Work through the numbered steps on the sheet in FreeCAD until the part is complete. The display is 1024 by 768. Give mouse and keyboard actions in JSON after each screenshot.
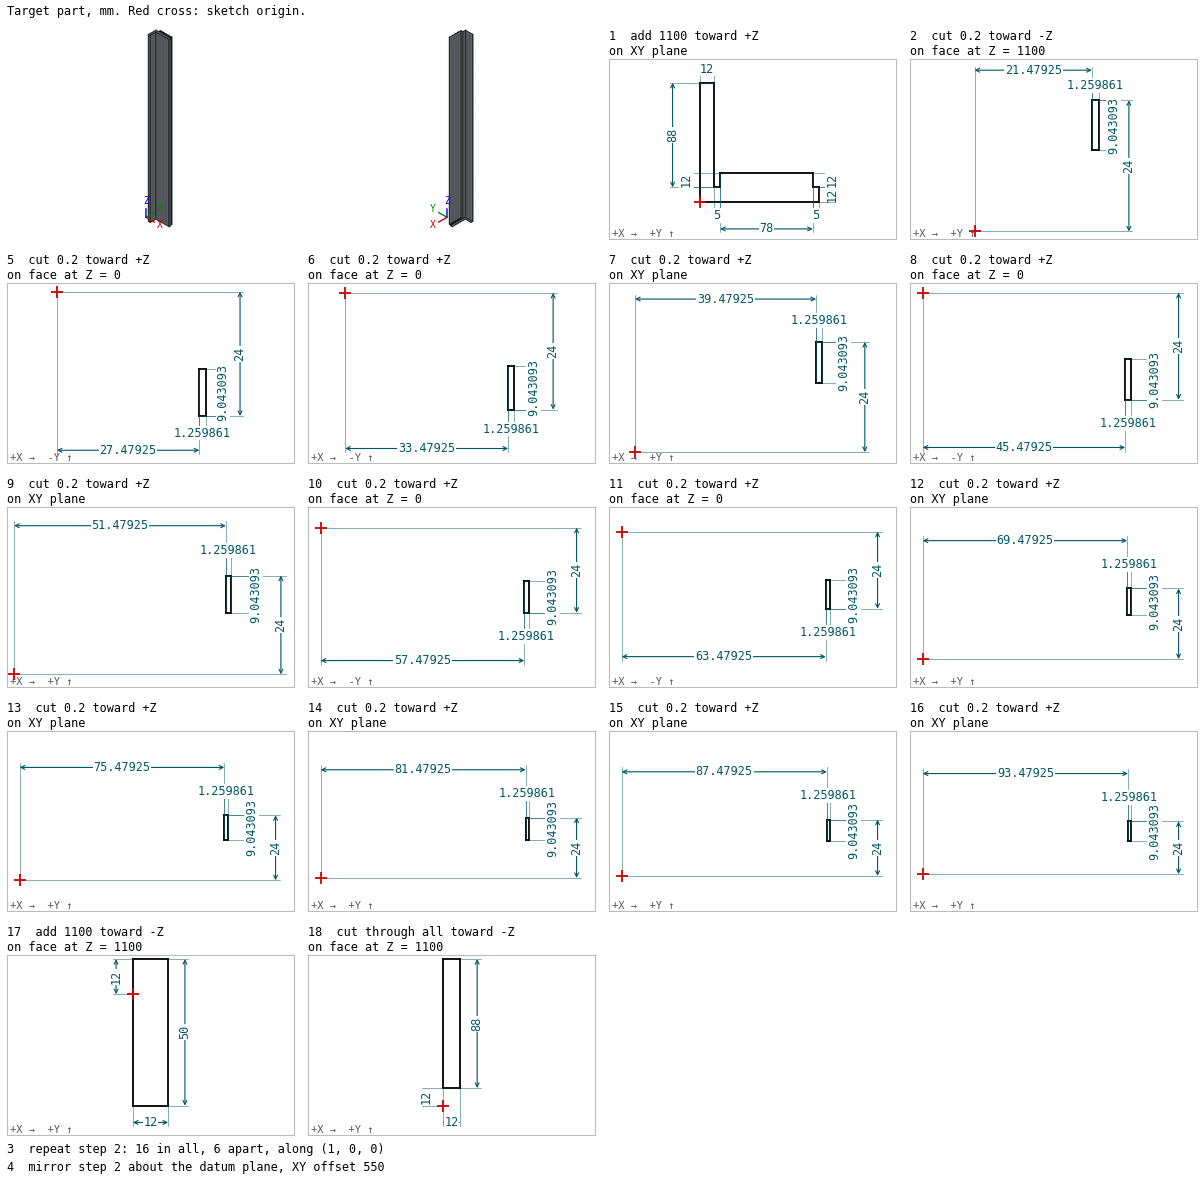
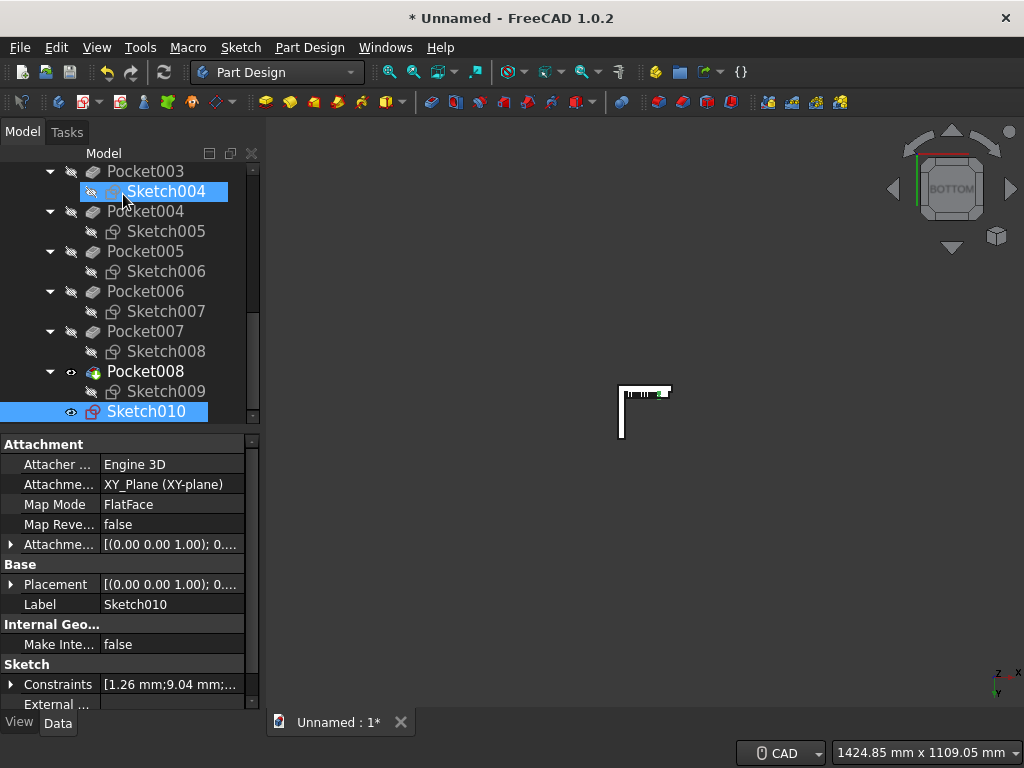
{"action": "left_click", "coordinate": [432, 102]}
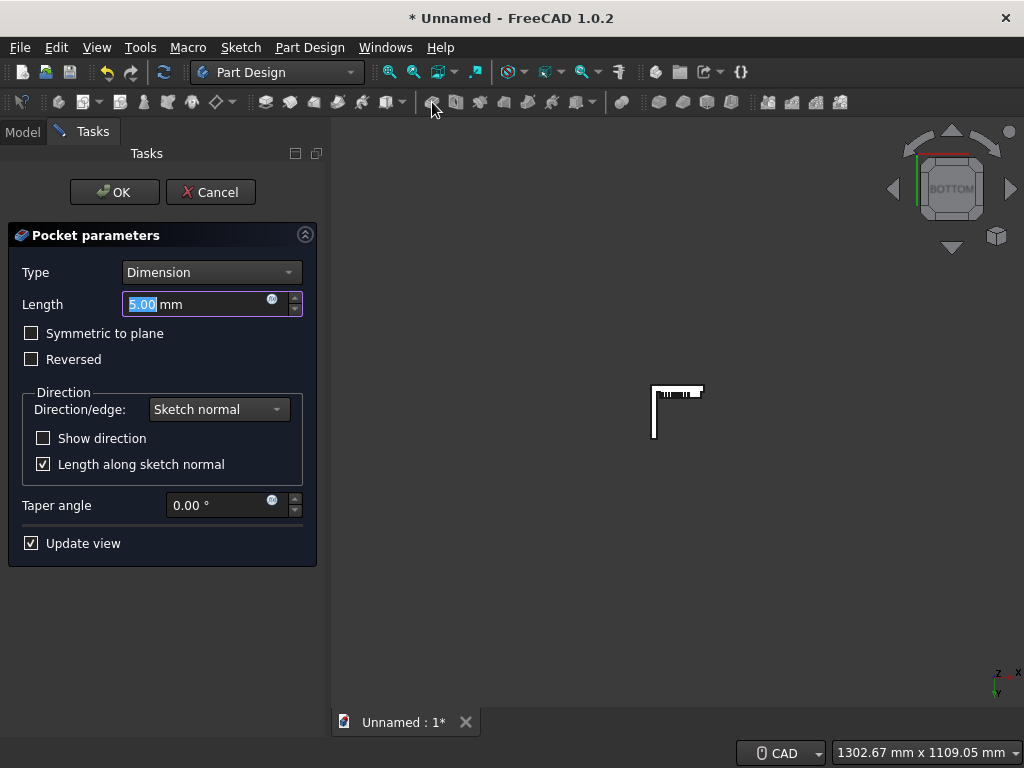
{"action": "type", "text": "0.2"}
{"action": "key", "text": "Tab"}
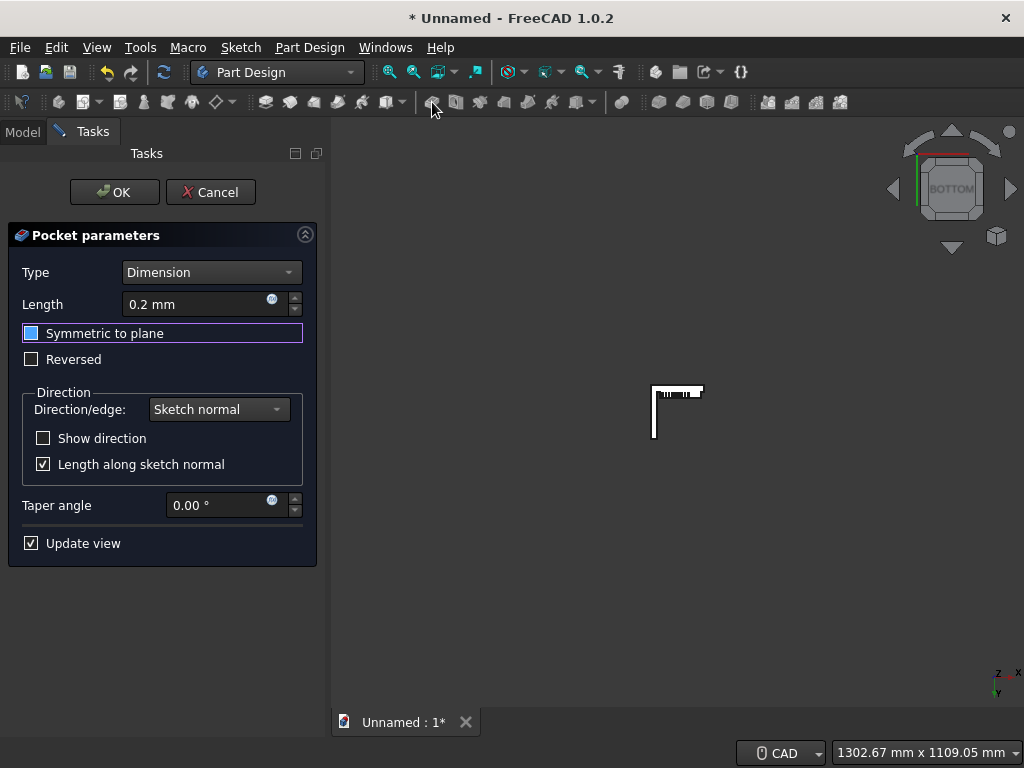
{"action": "left_click", "coordinate": [30, 359]}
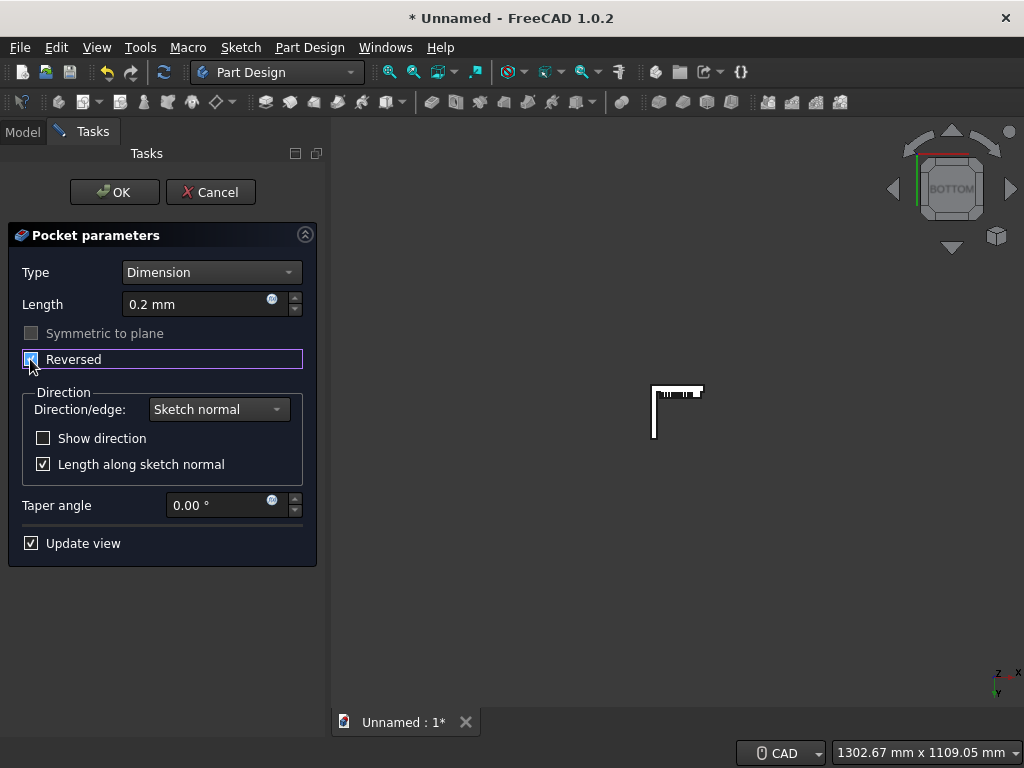
{"action": "left_click", "coordinate": [115, 192]}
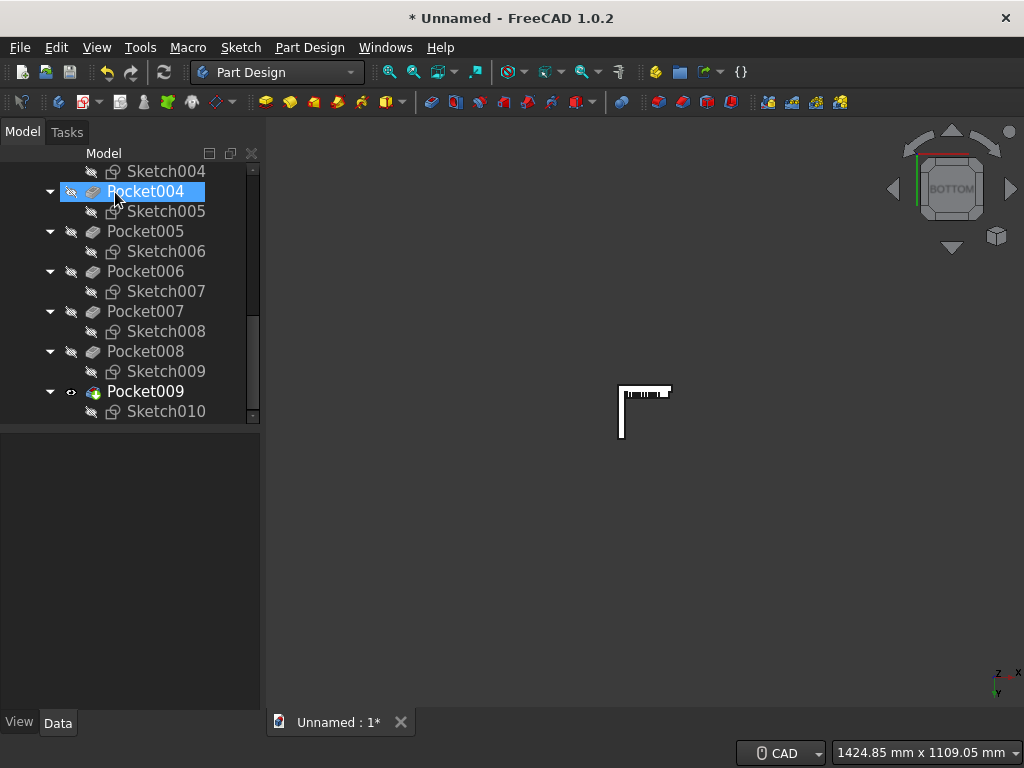
{"action": "left_click", "coordinate": [390, 72]}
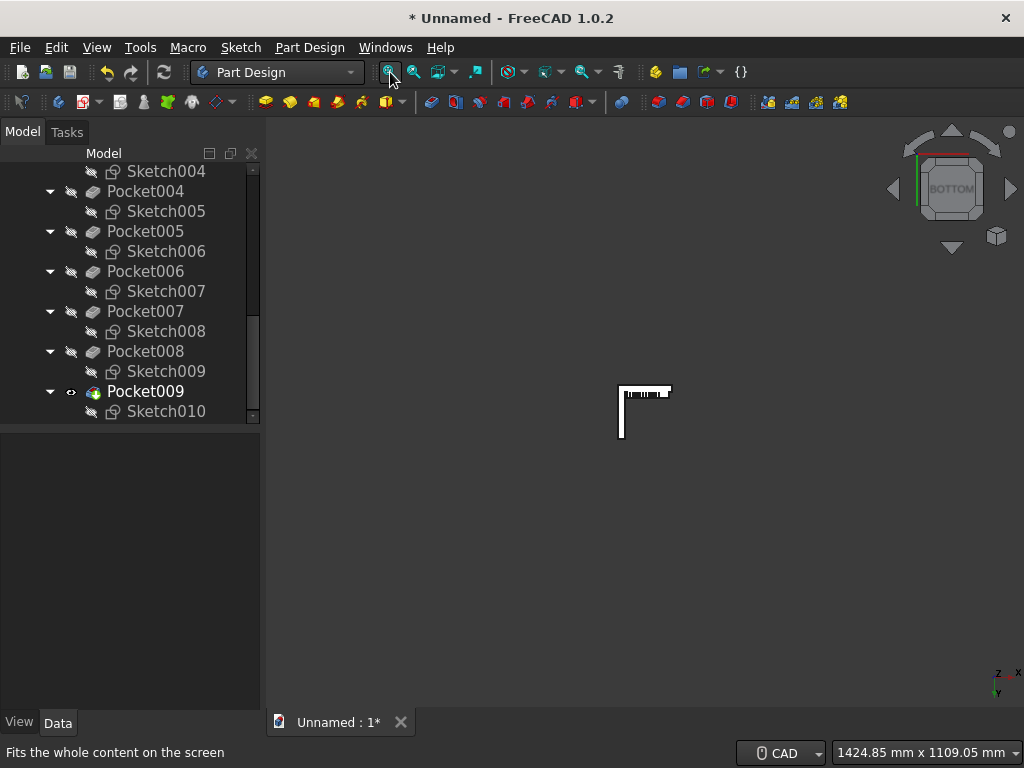
{"action": "left_click", "coordinate": [84, 102]}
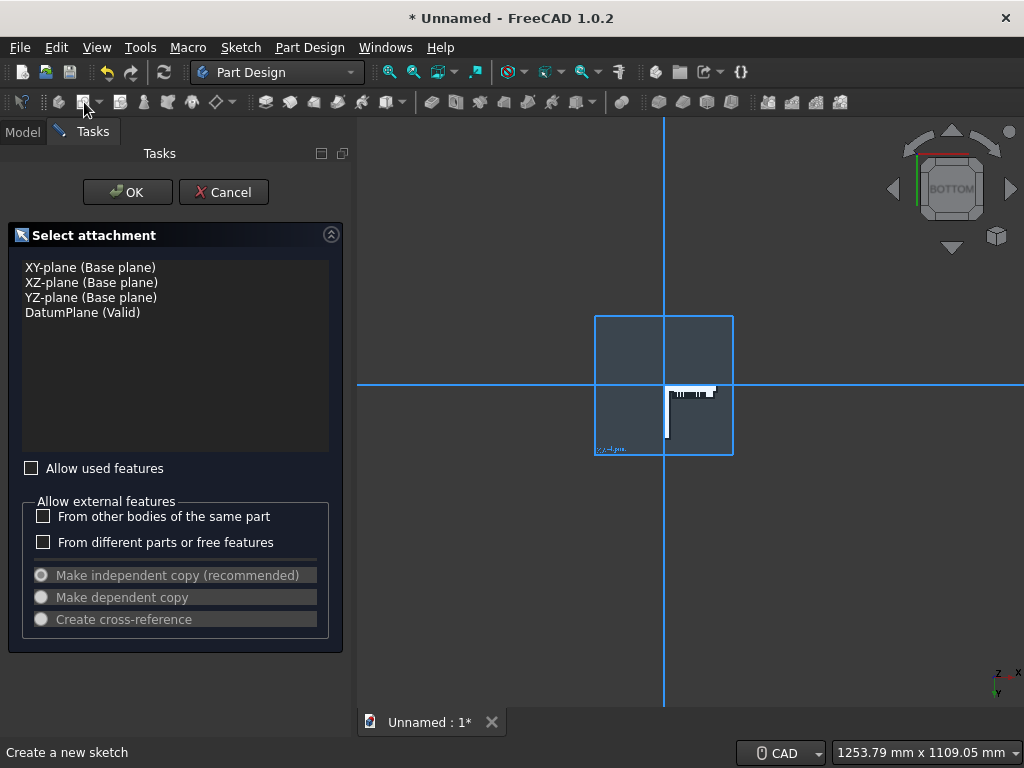
{"action": "left_click", "coordinate": [82, 268]}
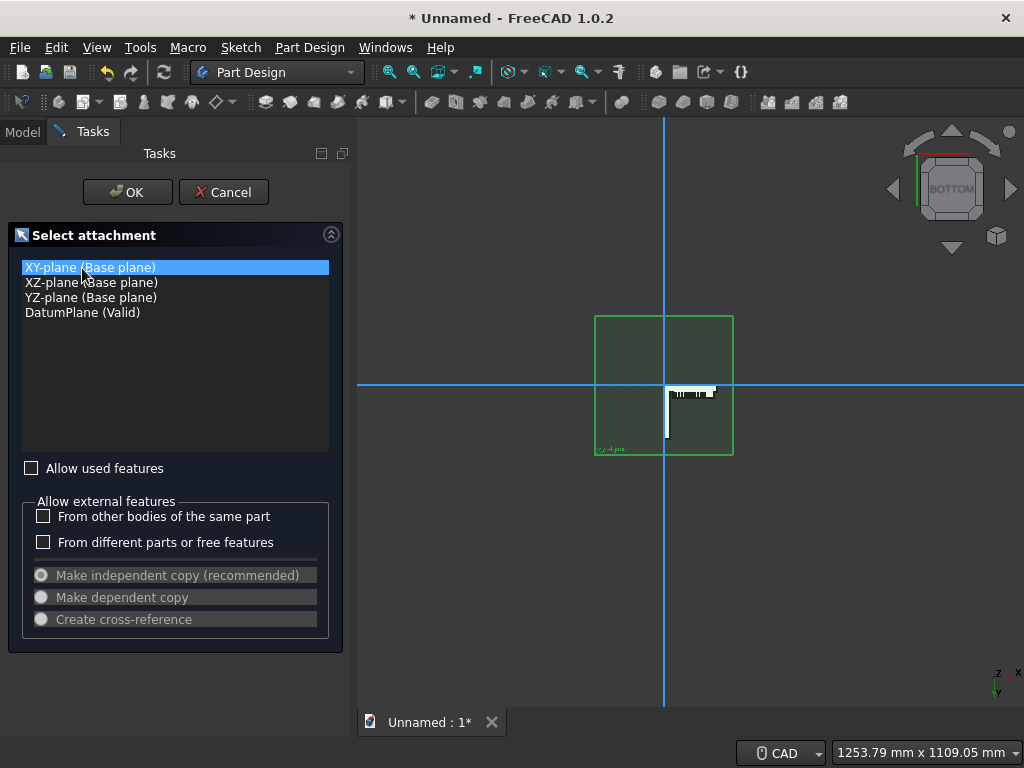
{"action": "left_click", "coordinate": [128, 192]}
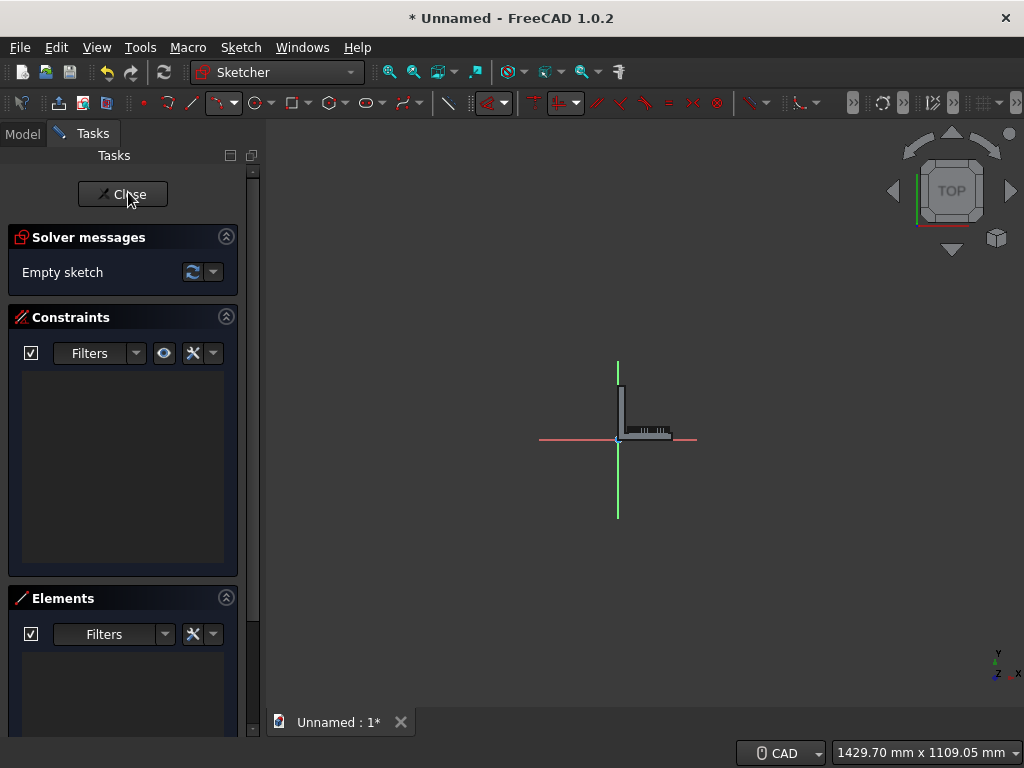
{"action": "left_click", "coordinate": [108, 104]}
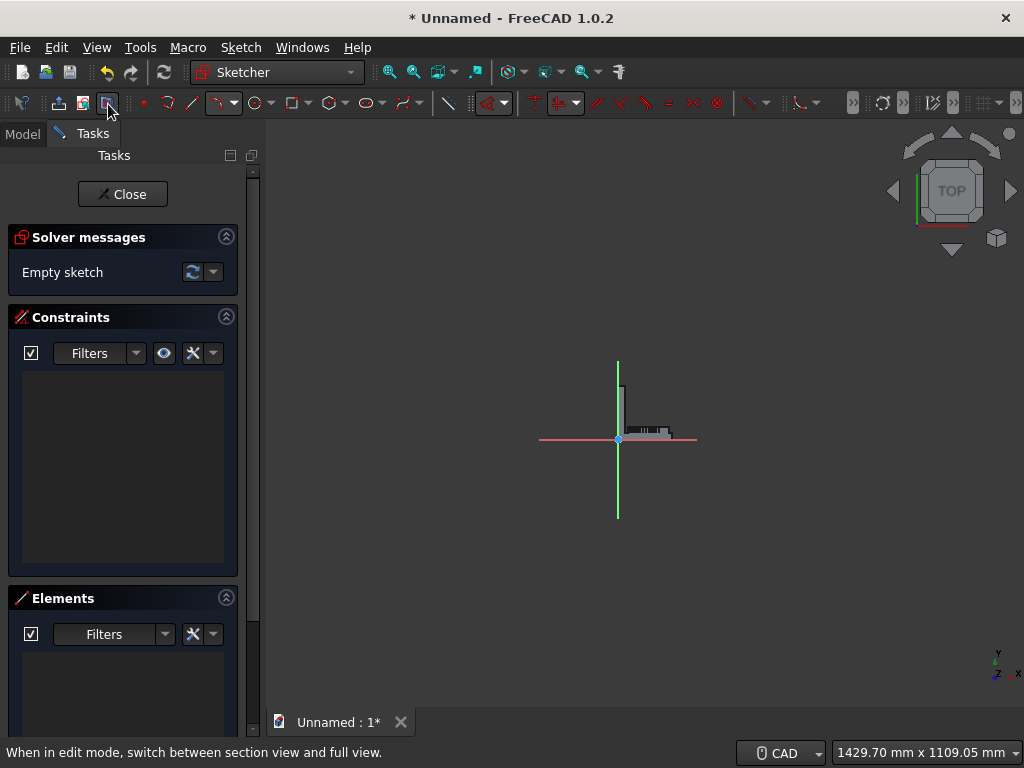
{"action": "scroll", "coordinate": [667, 430], "scroll_direction": "up", "scroll_amount": 15}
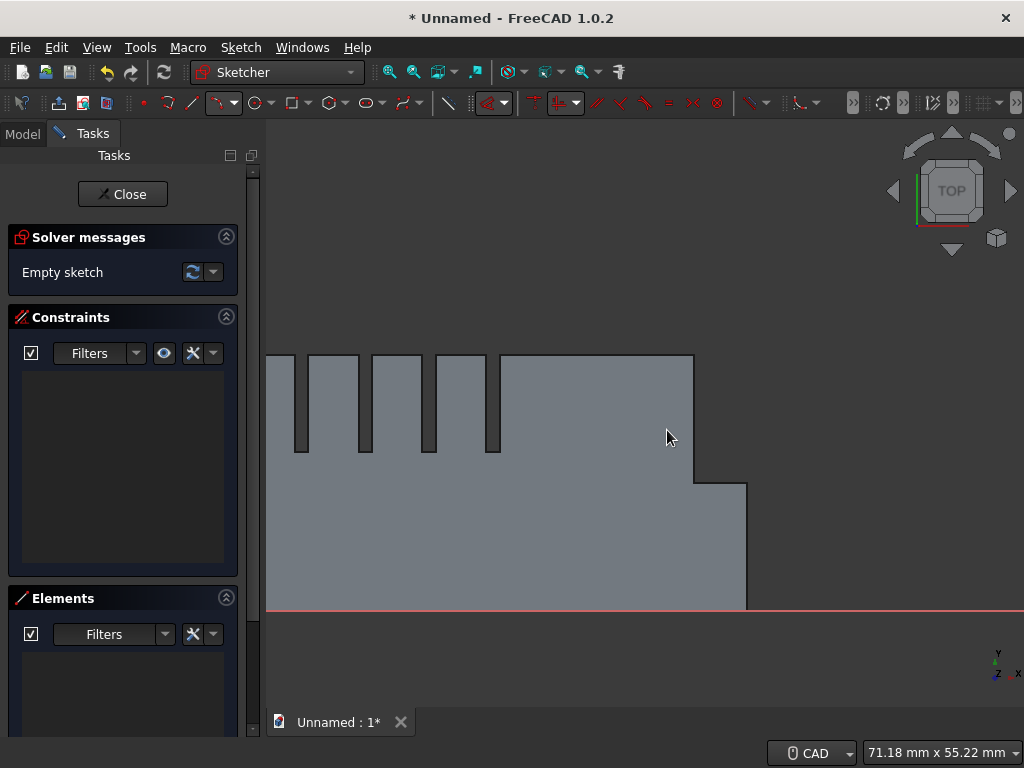
{"action": "scroll", "coordinate": [551, 400], "scroll_direction": "up", "scroll_amount": 7}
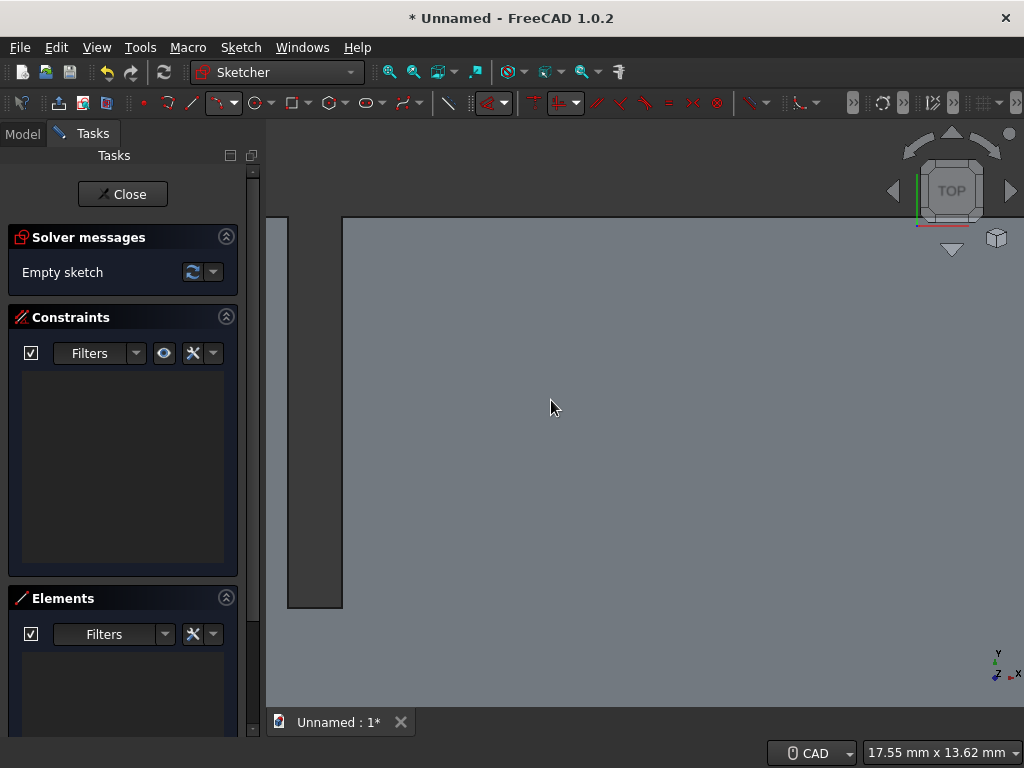
{"action": "left_click", "coordinate": [292, 104]}